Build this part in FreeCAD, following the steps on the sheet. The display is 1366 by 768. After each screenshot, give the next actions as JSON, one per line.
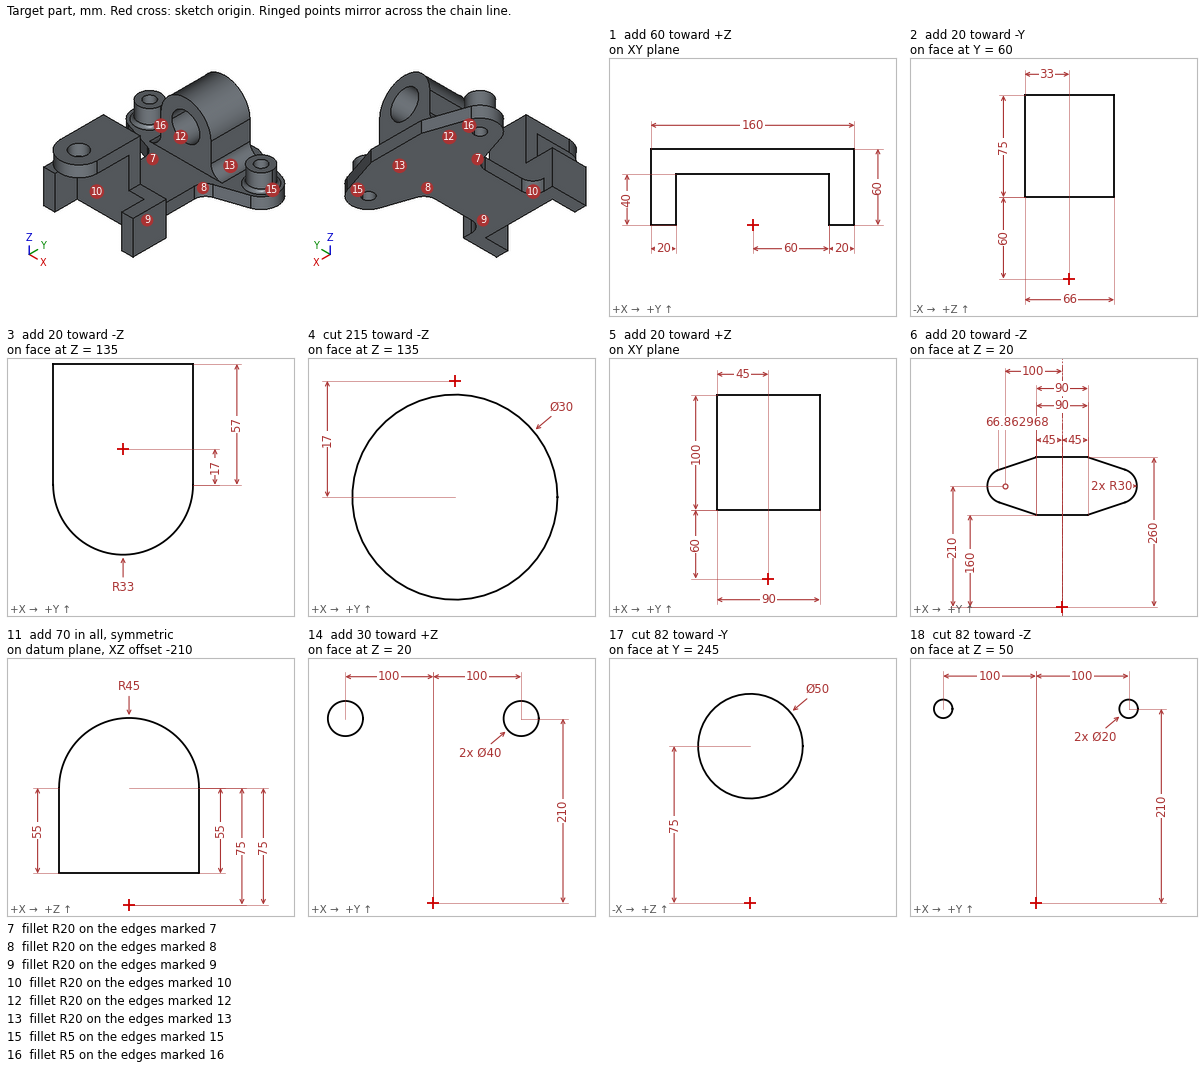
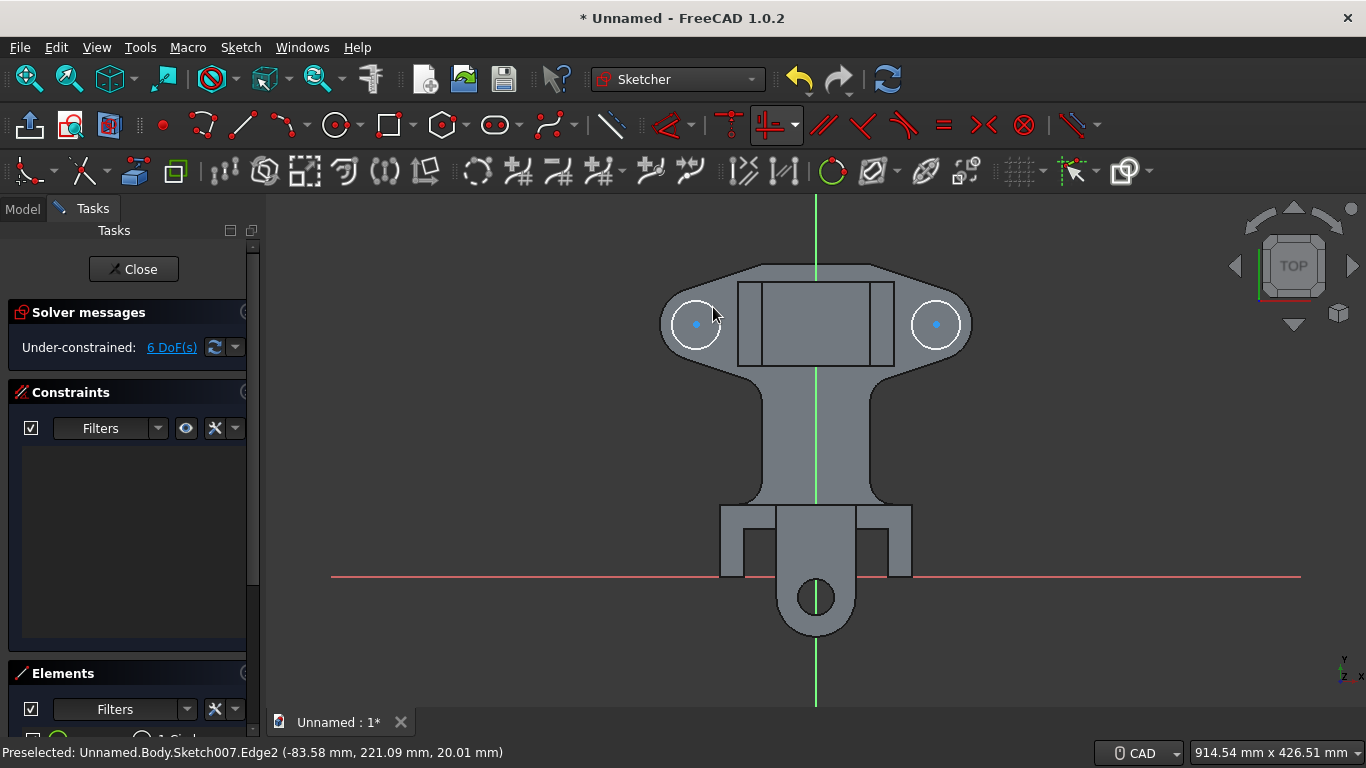
{"action": "left_click", "coordinate": [953, 308]}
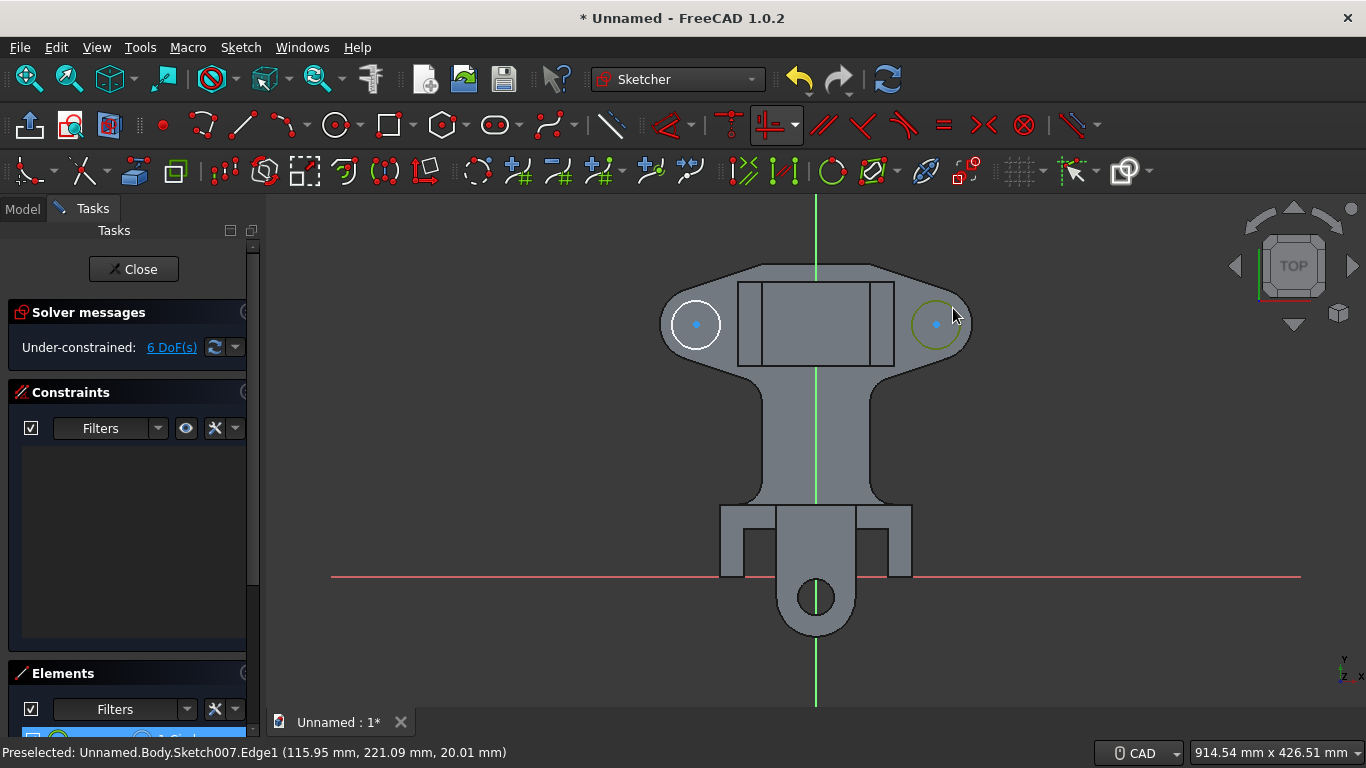
{"action": "left_click", "coordinate": [713, 308]}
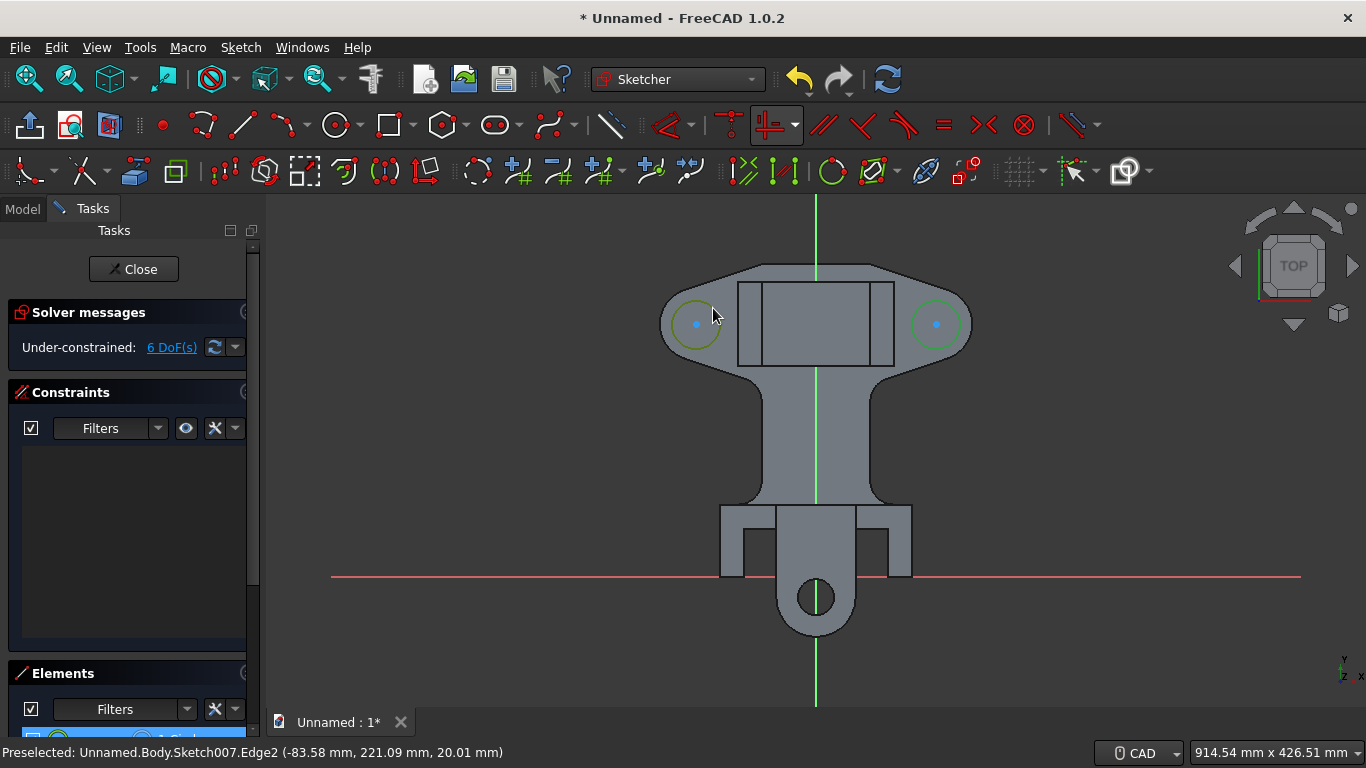
{"action": "key", "text": "e"}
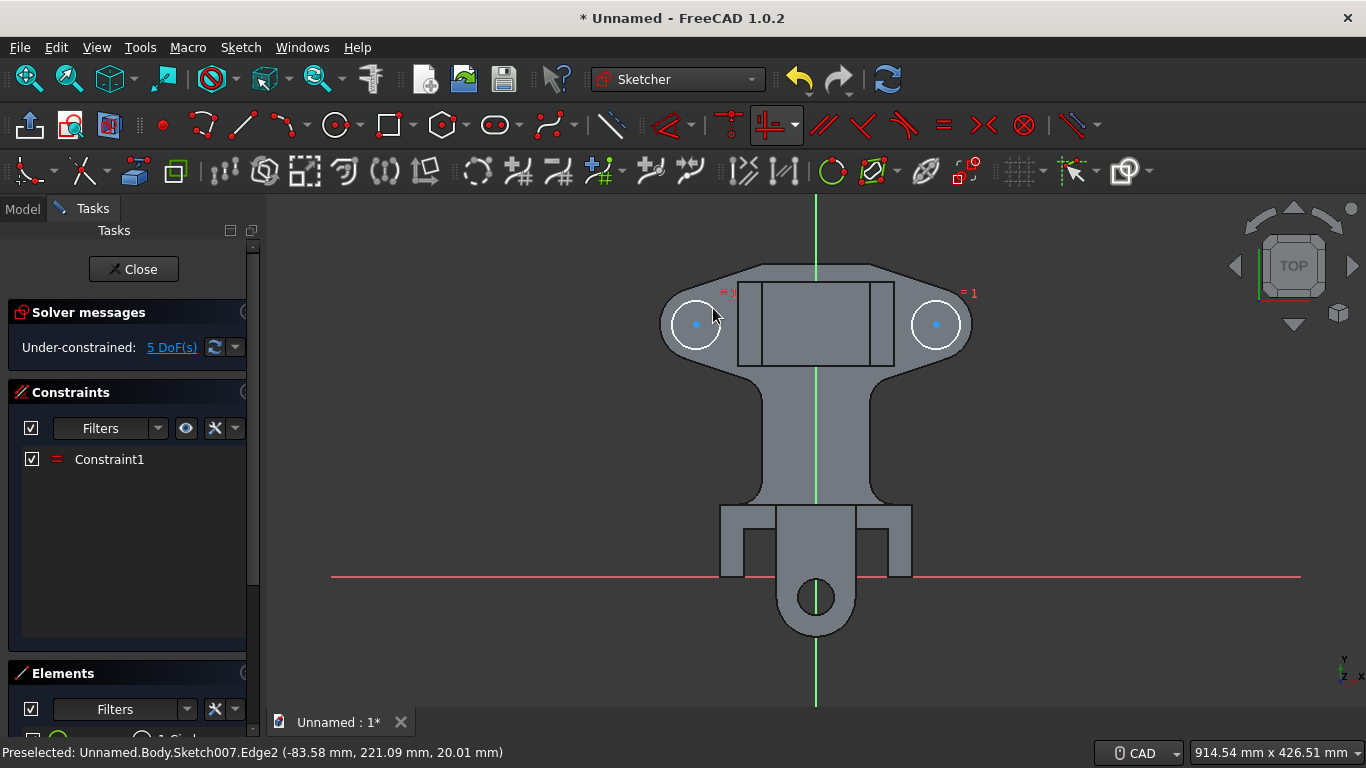
{"action": "left_click", "coordinate": [936, 325]}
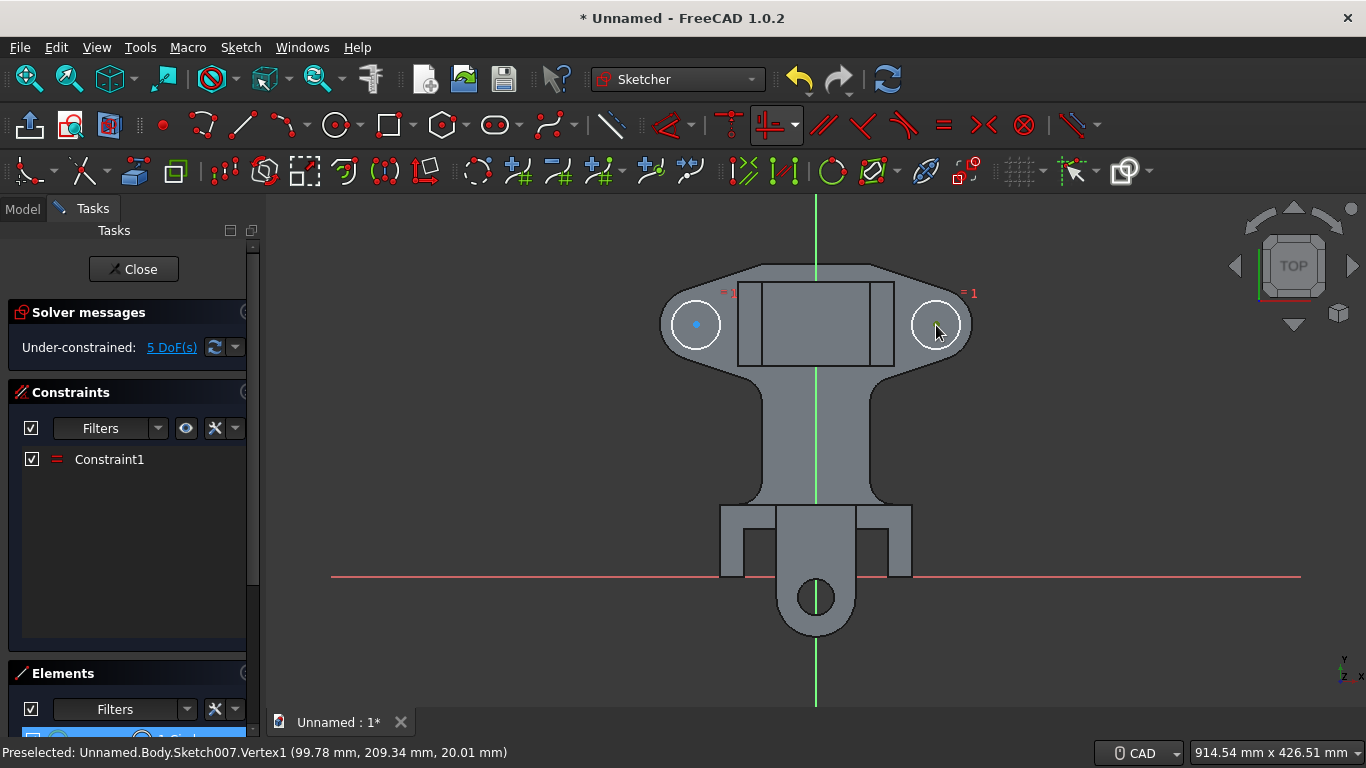
{"action": "left_click", "coordinate": [696, 325]}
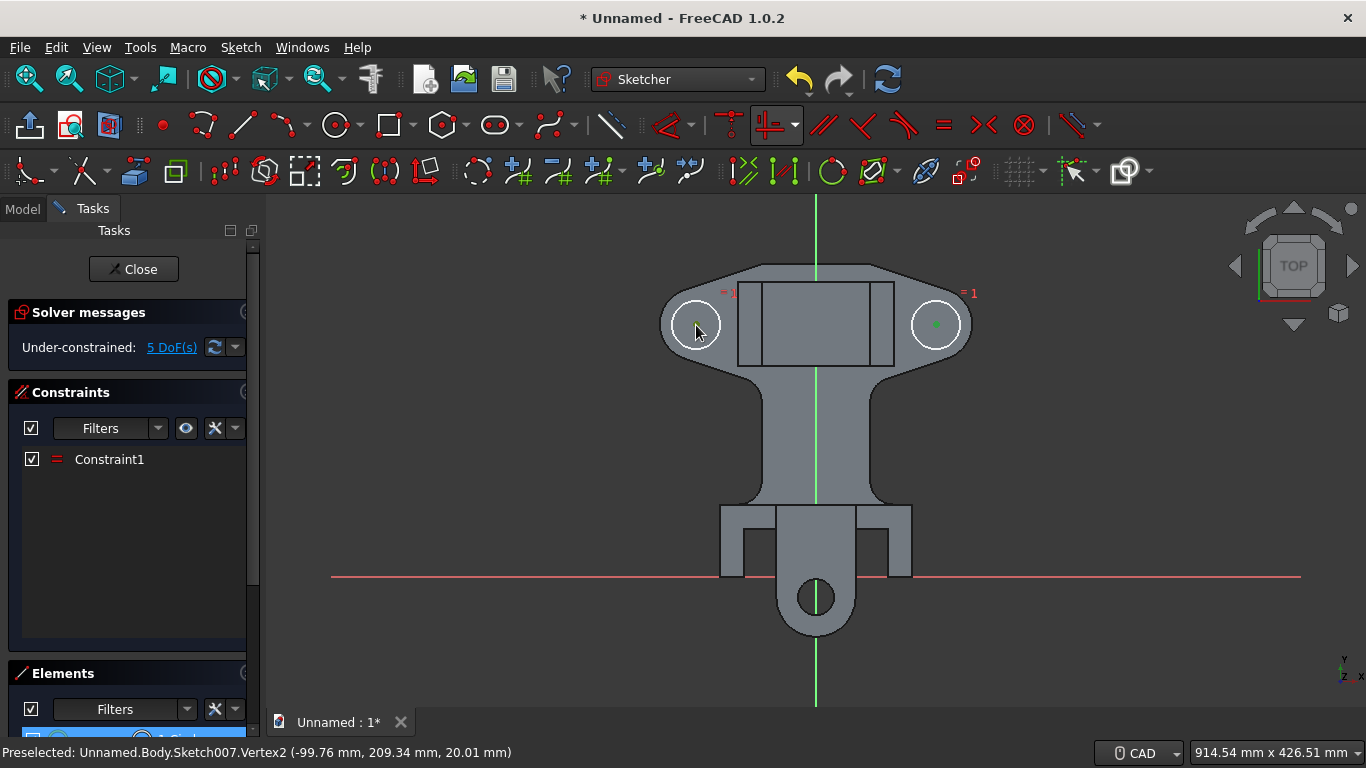
{"action": "key", "text": "h"}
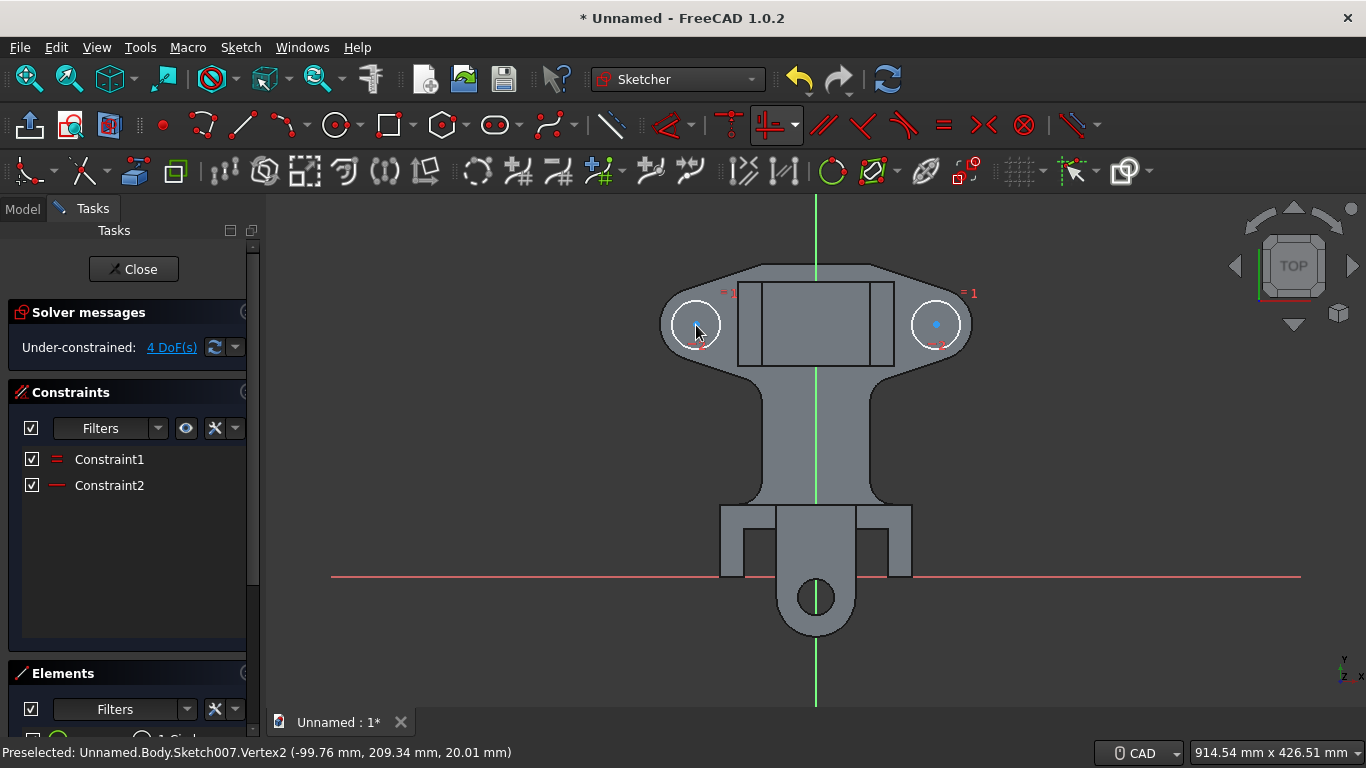
{"action": "key", "text": "d"}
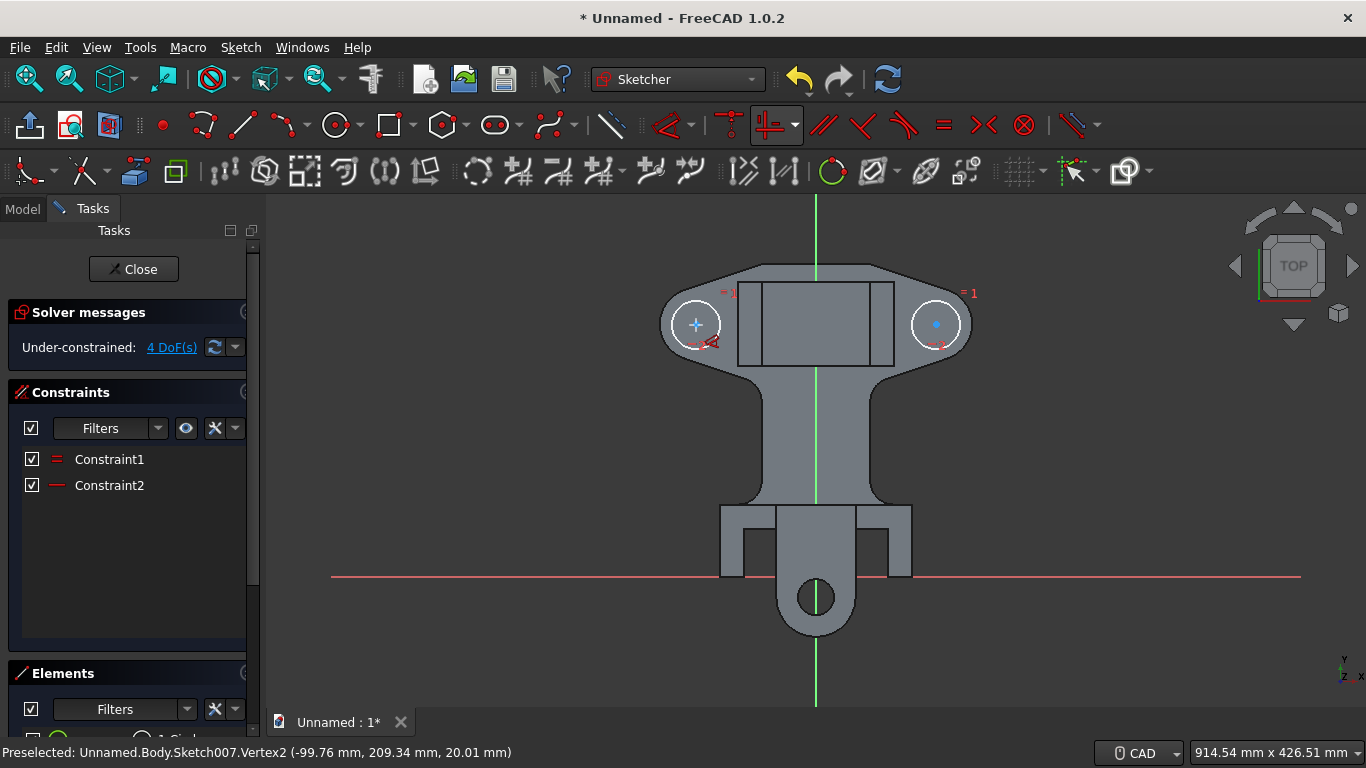
{"action": "left_click", "coordinate": [953, 308]}
{"action": "left_click", "coordinate": [976, 285]}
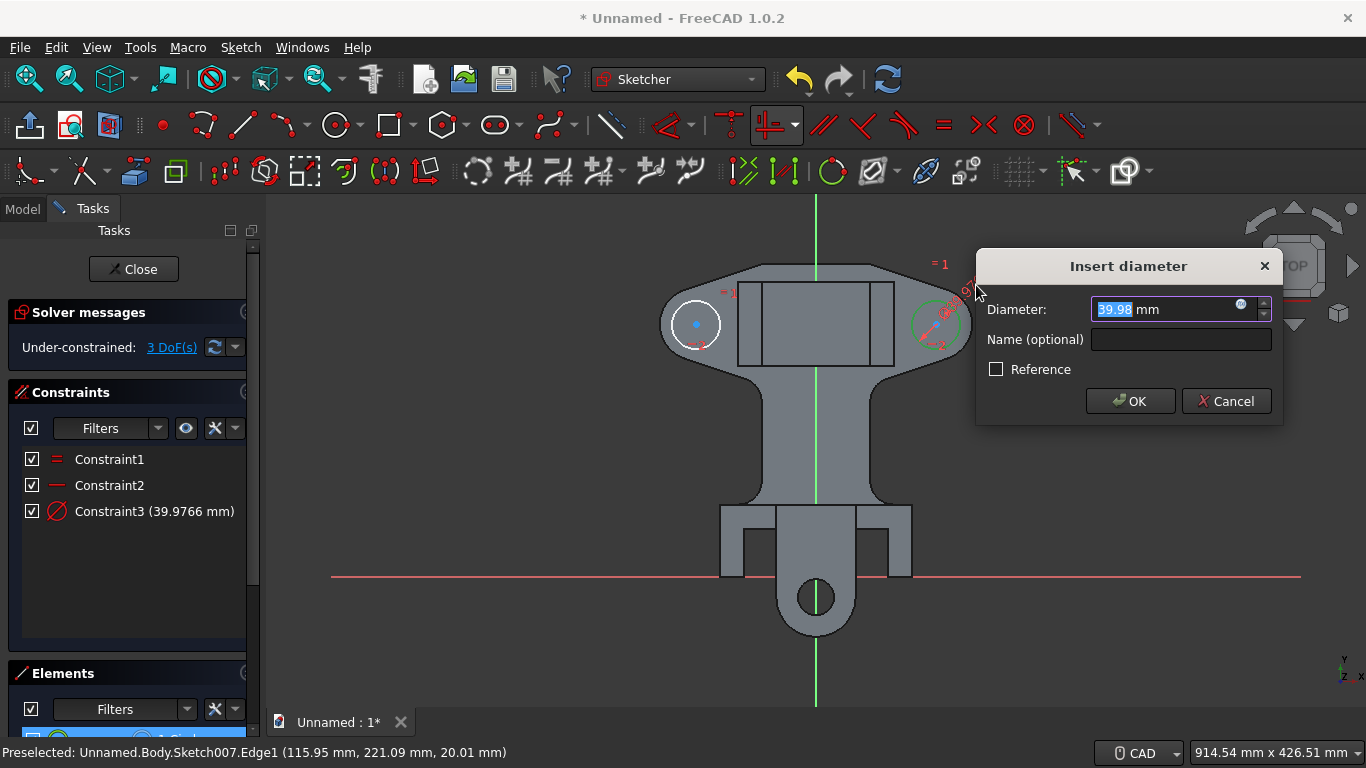
{"action": "type", "text": "40"}
{"action": "key", "text": "Return"}